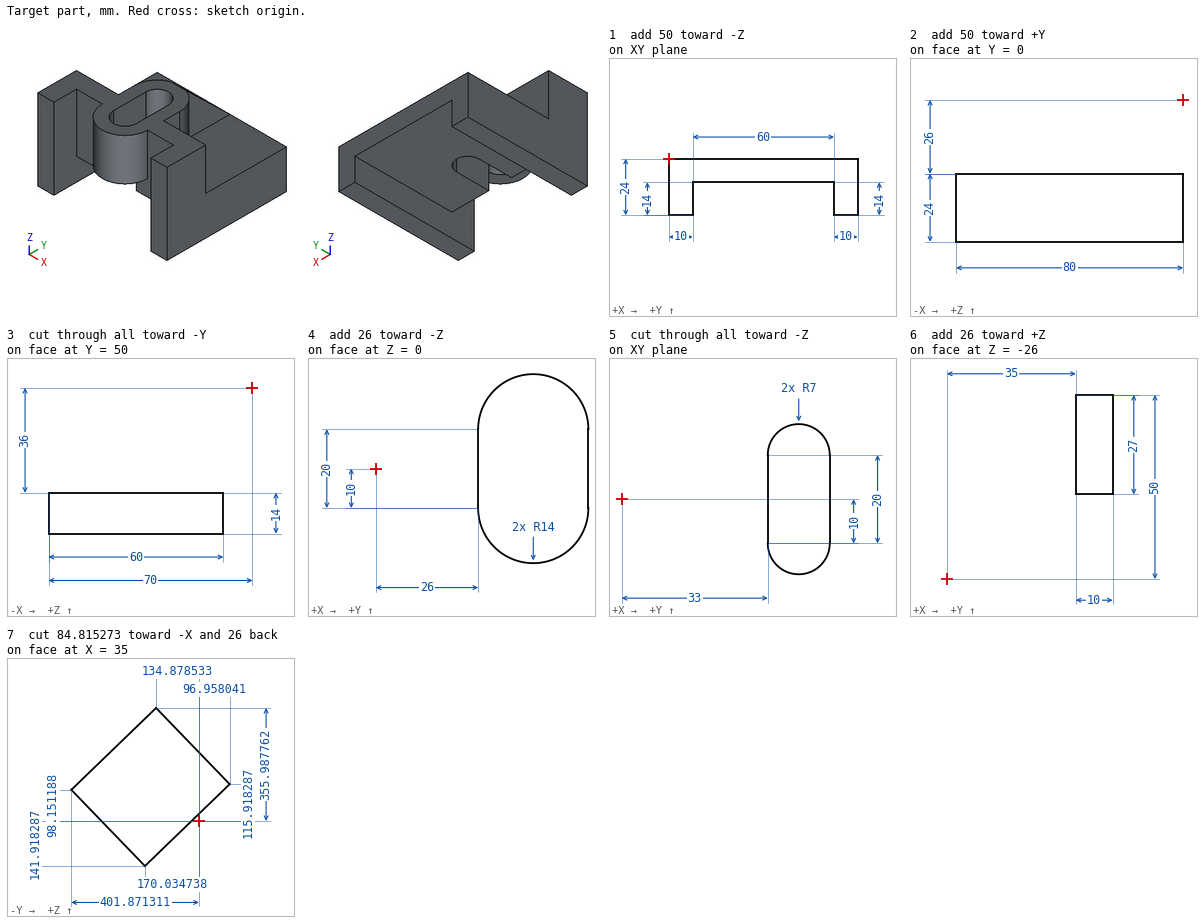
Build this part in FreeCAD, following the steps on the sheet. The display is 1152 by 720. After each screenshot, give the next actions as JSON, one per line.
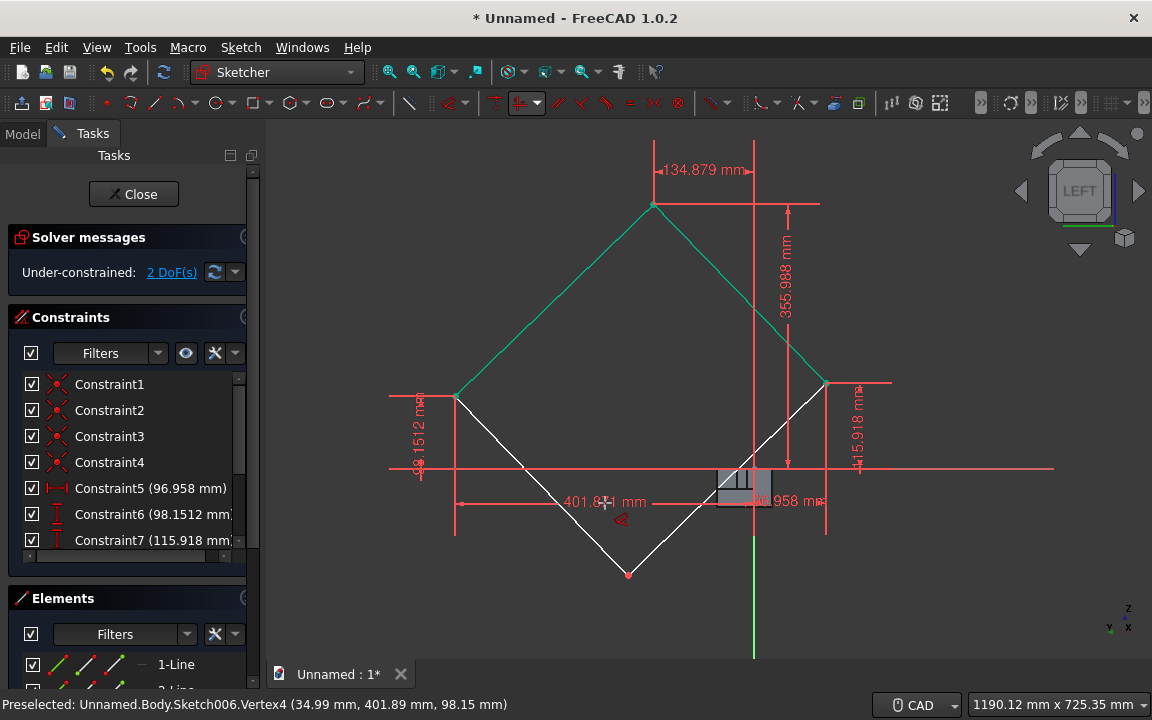
{"action": "left_click", "coordinate": [628, 576]}
{"action": "left_click", "coordinate": [691, 610]}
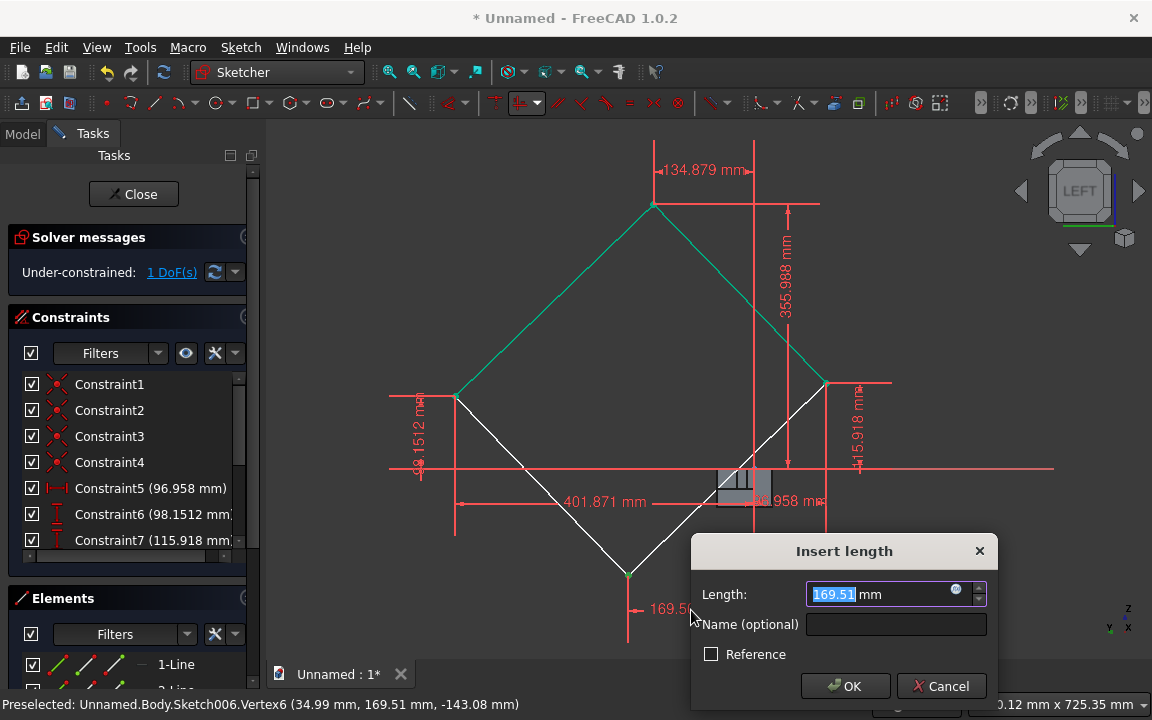
{"action": "type", "text": "170.034738"}
{"action": "key", "text": "Return"}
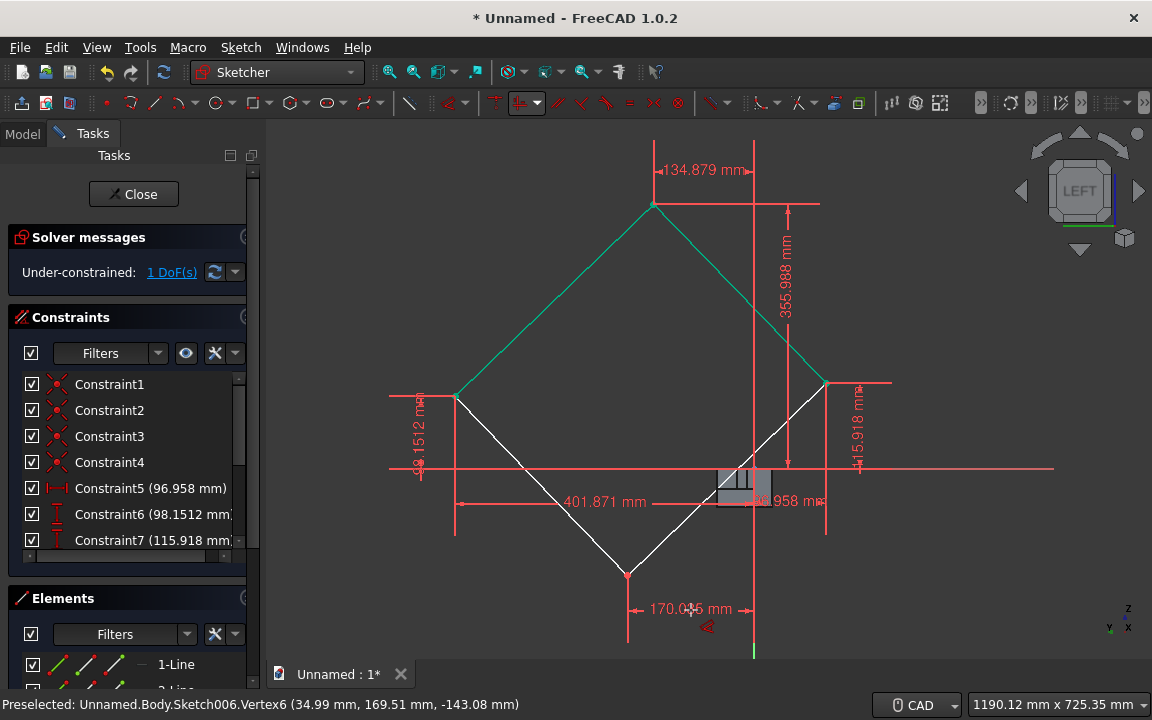
{"action": "left_click", "coordinate": [628, 576]}
{"action": "left_click", "coordinate": [788, 547]}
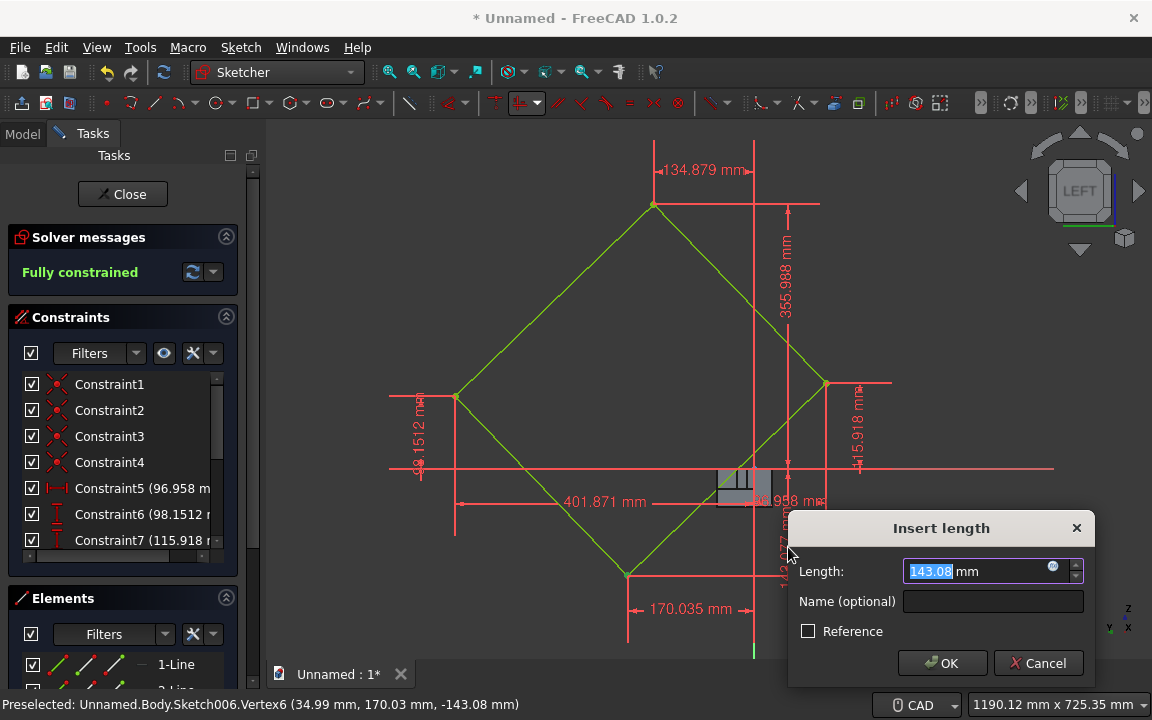
{"action": "type", "text": "141.918287"}
{"action": "key", "text": "Return"}
{"action": "key", "text": "Escape"}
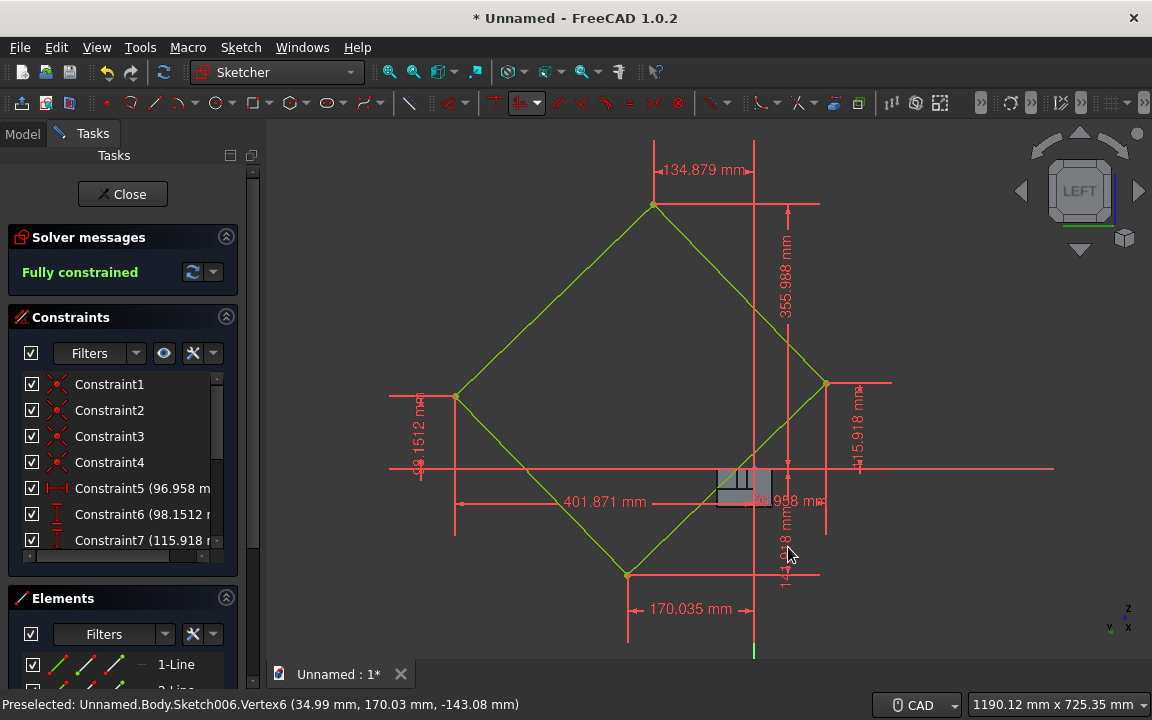
{"action": "left_click", "coordinate": [123, 194]}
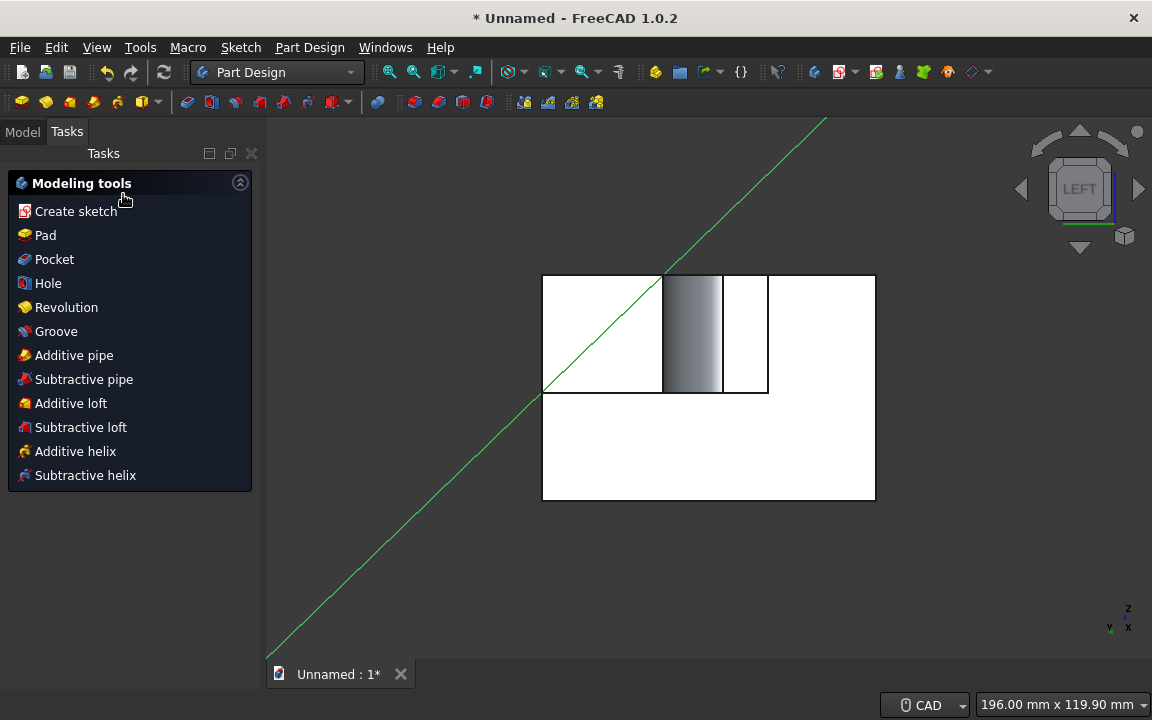
{"action": "left_click", "coordinate": [188, 102]}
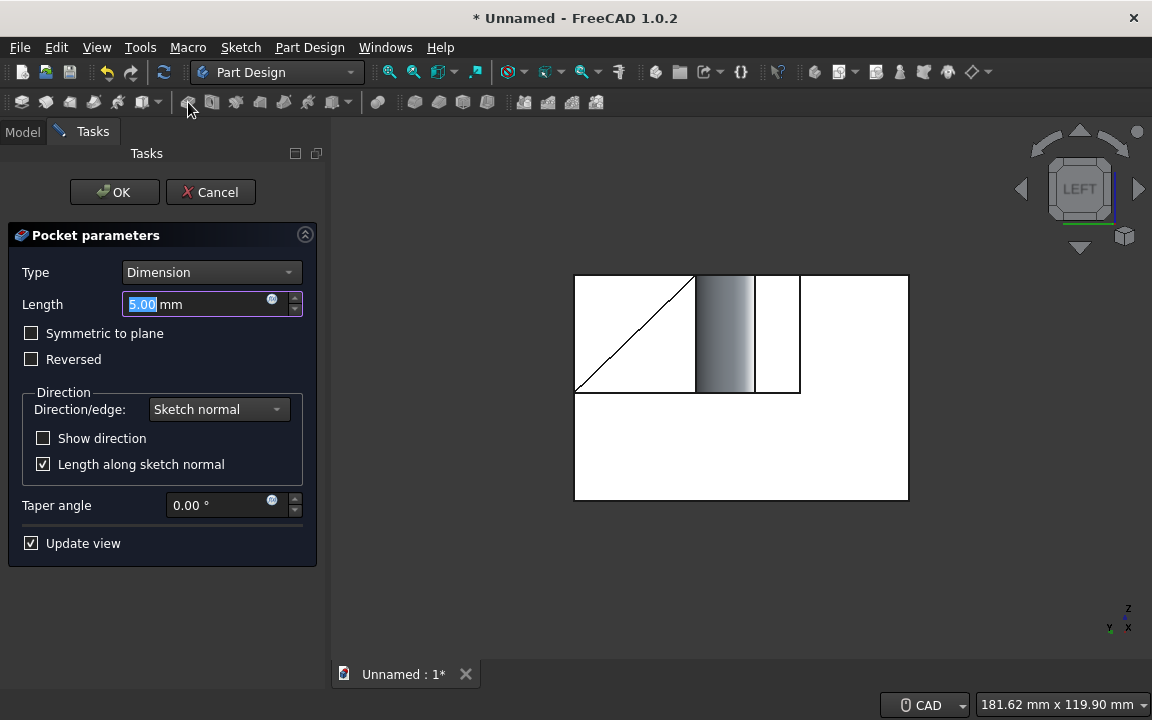
{"action": "left_click", "coordinate": [212, 272]}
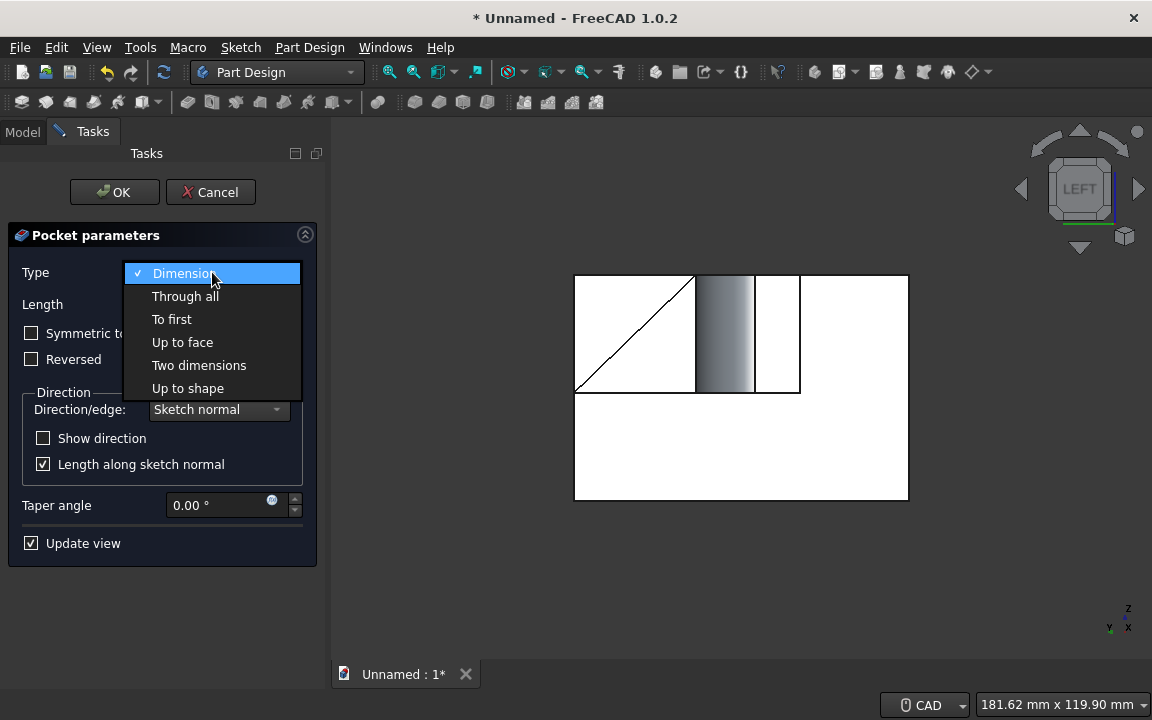
{"action": "left_click", "coordinate": [212, 366]}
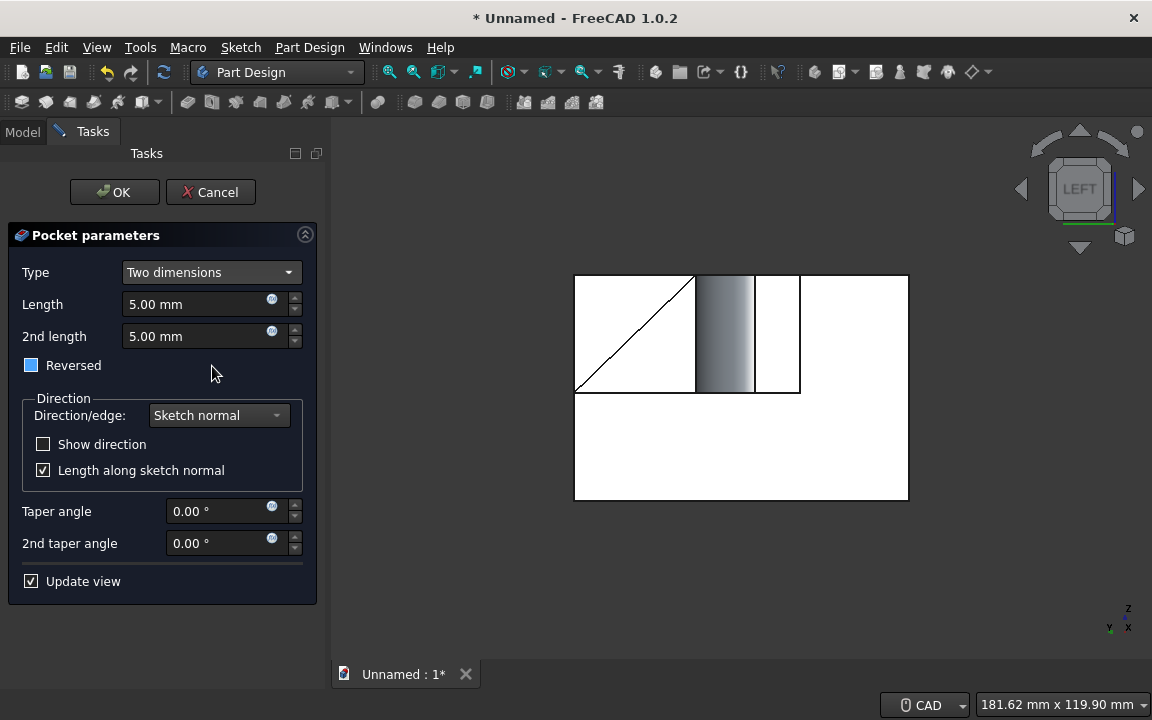
{"action": "triple_click", "coordinate": [204, 304]}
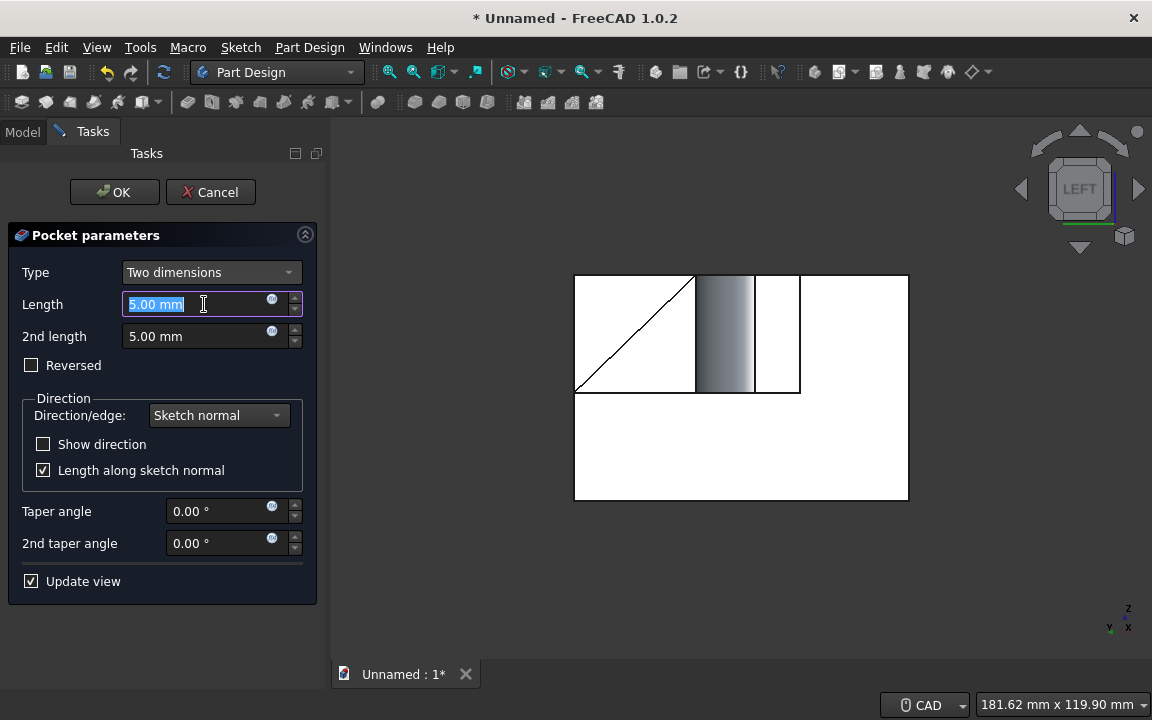
{"action": "type", "text": "84.815273"}
{"action": "key", "text": "Tab"}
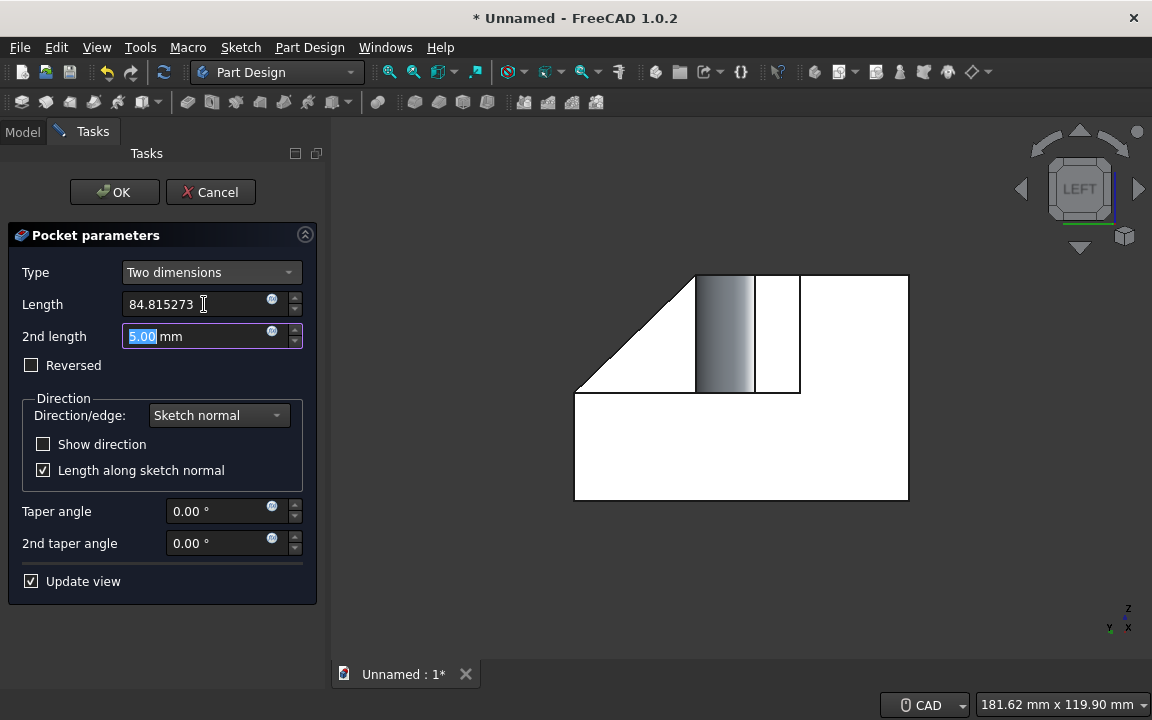
{"action": "type", "text": "26"}
{"action": "key", "text": "Tab"}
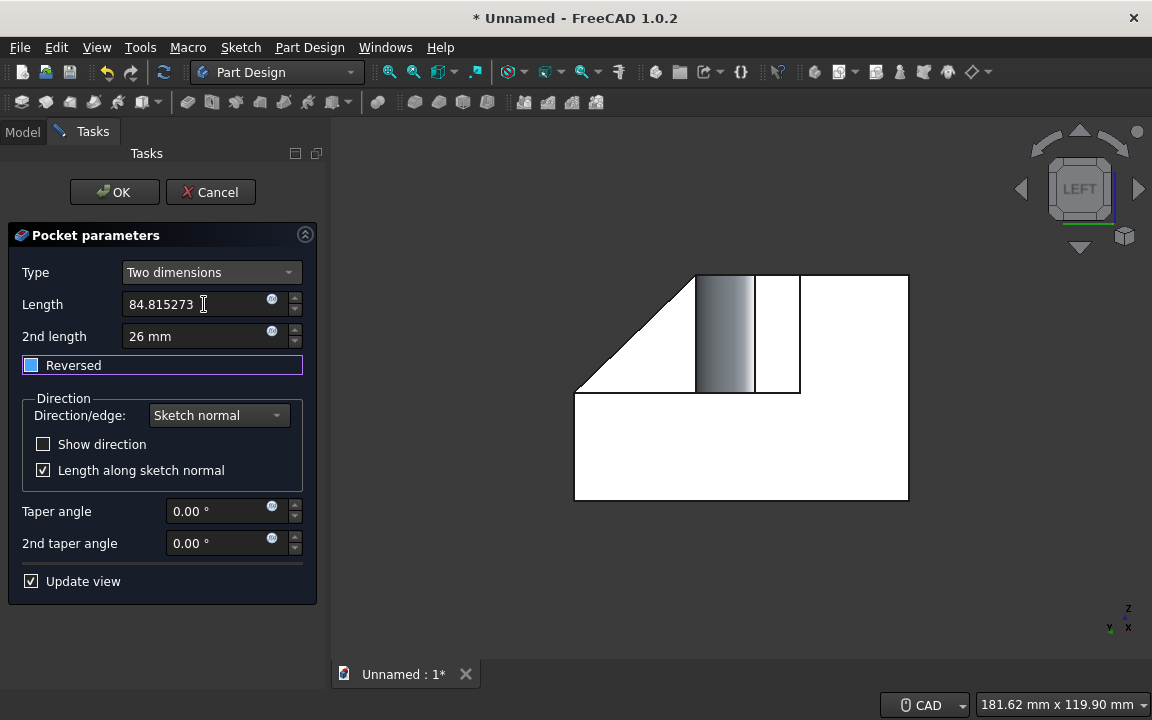
{"action": "left_click", "coordinate": [30, 365]}